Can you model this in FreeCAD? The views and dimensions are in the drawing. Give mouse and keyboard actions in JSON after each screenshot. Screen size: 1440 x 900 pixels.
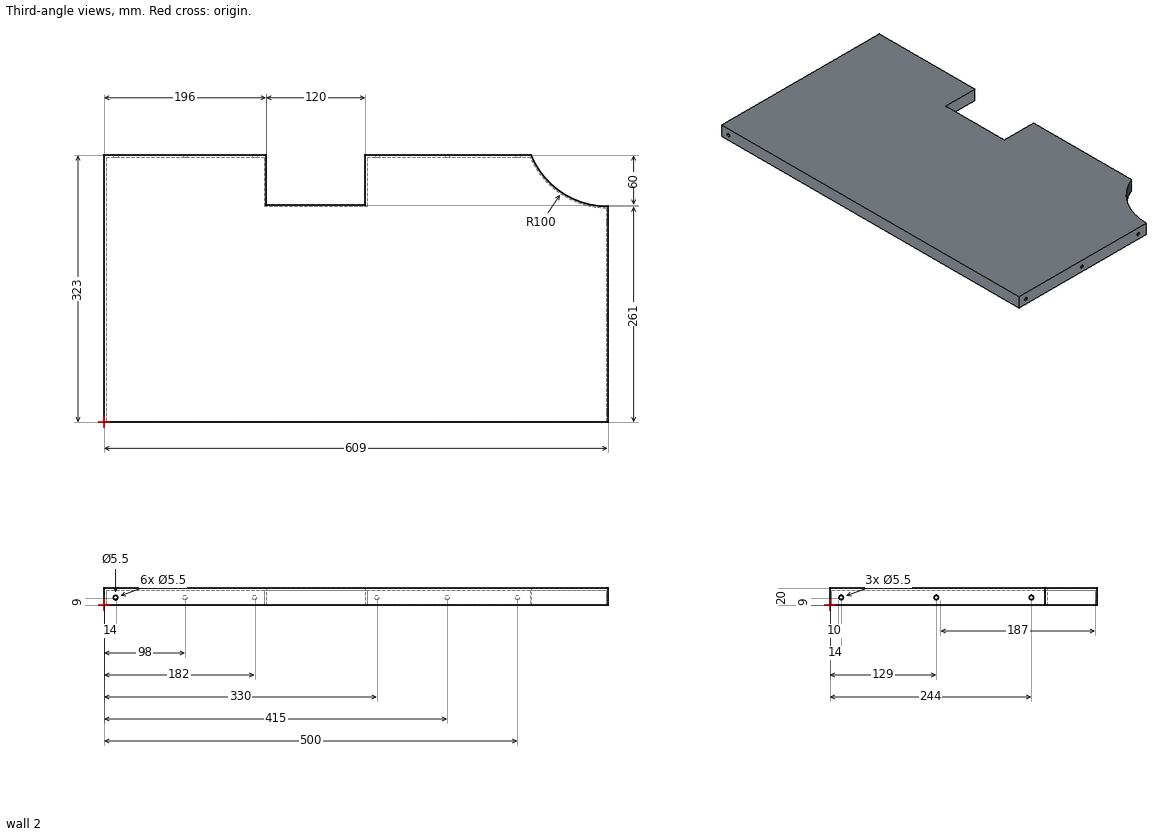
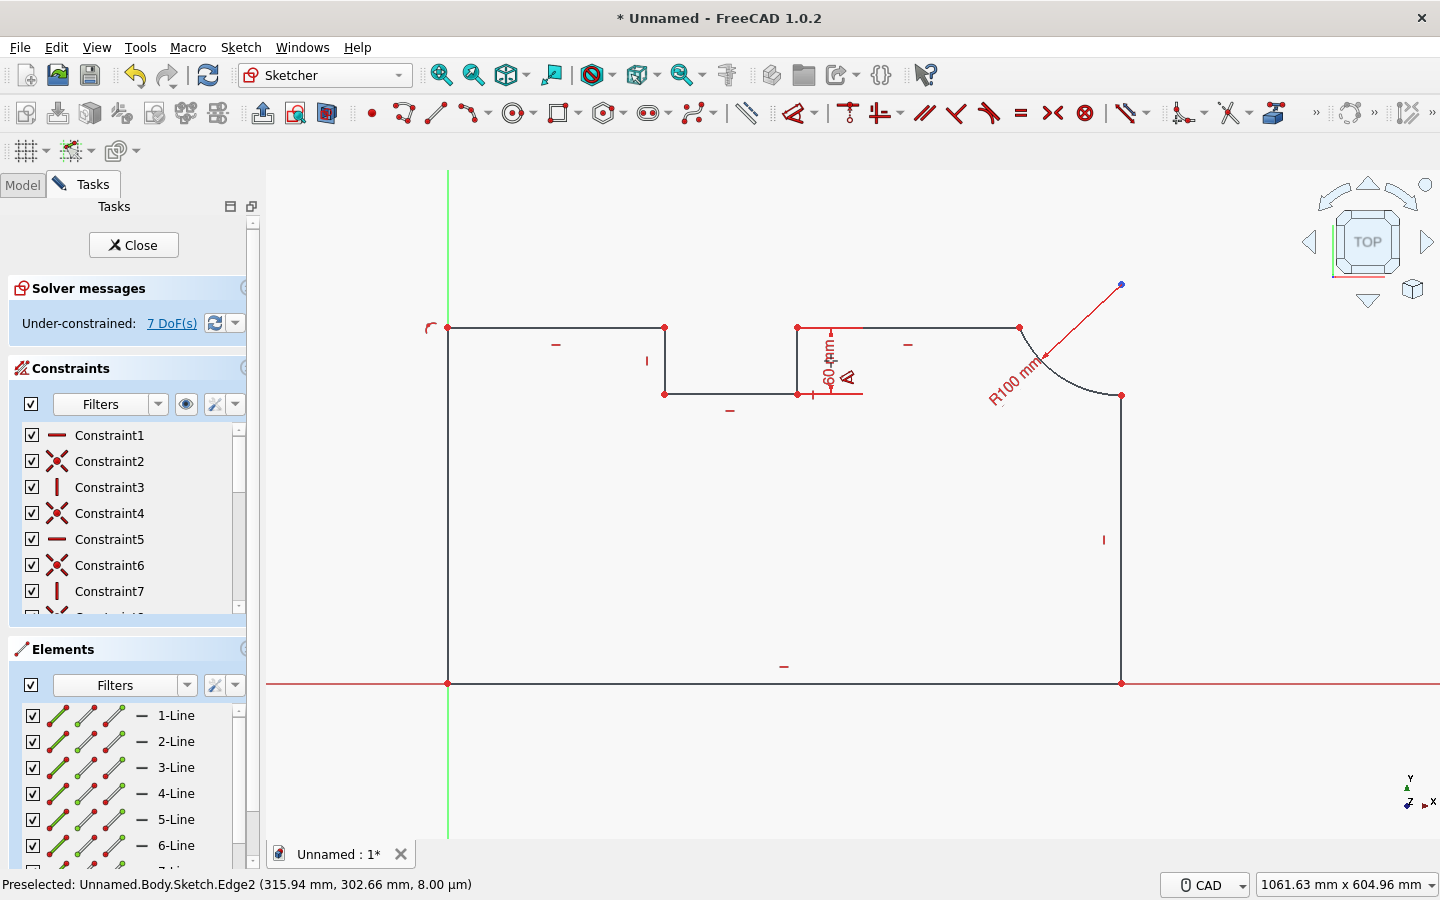
{"action": "left_click", "coordinate": [665, 374]}
{"action": "left_click", "coordinate": [631, 361]}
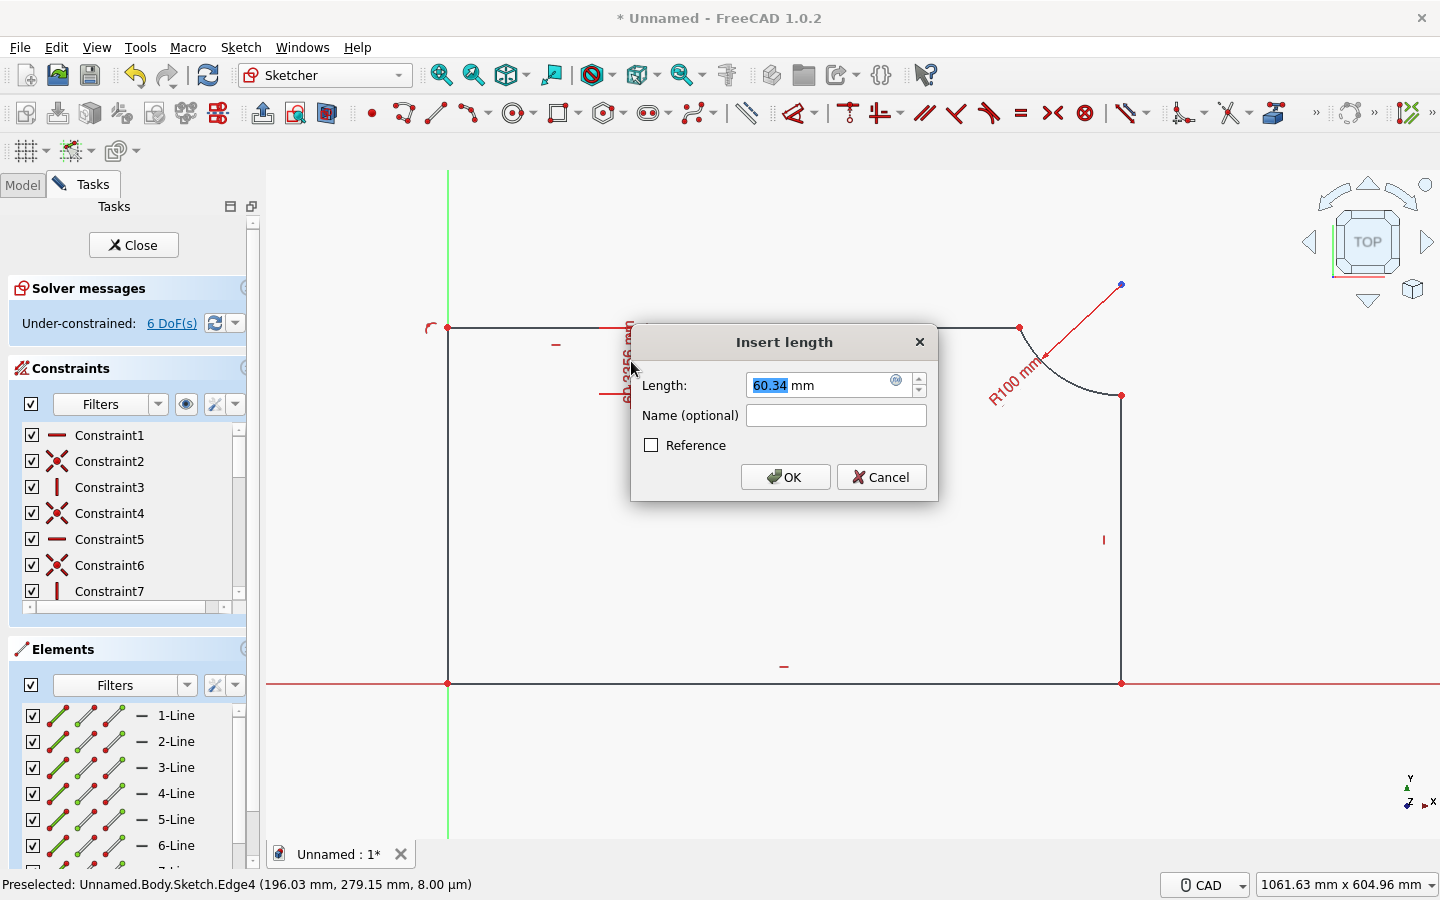
{"action": "type", "text": "60"}
{"action": "key", "text": "Return"}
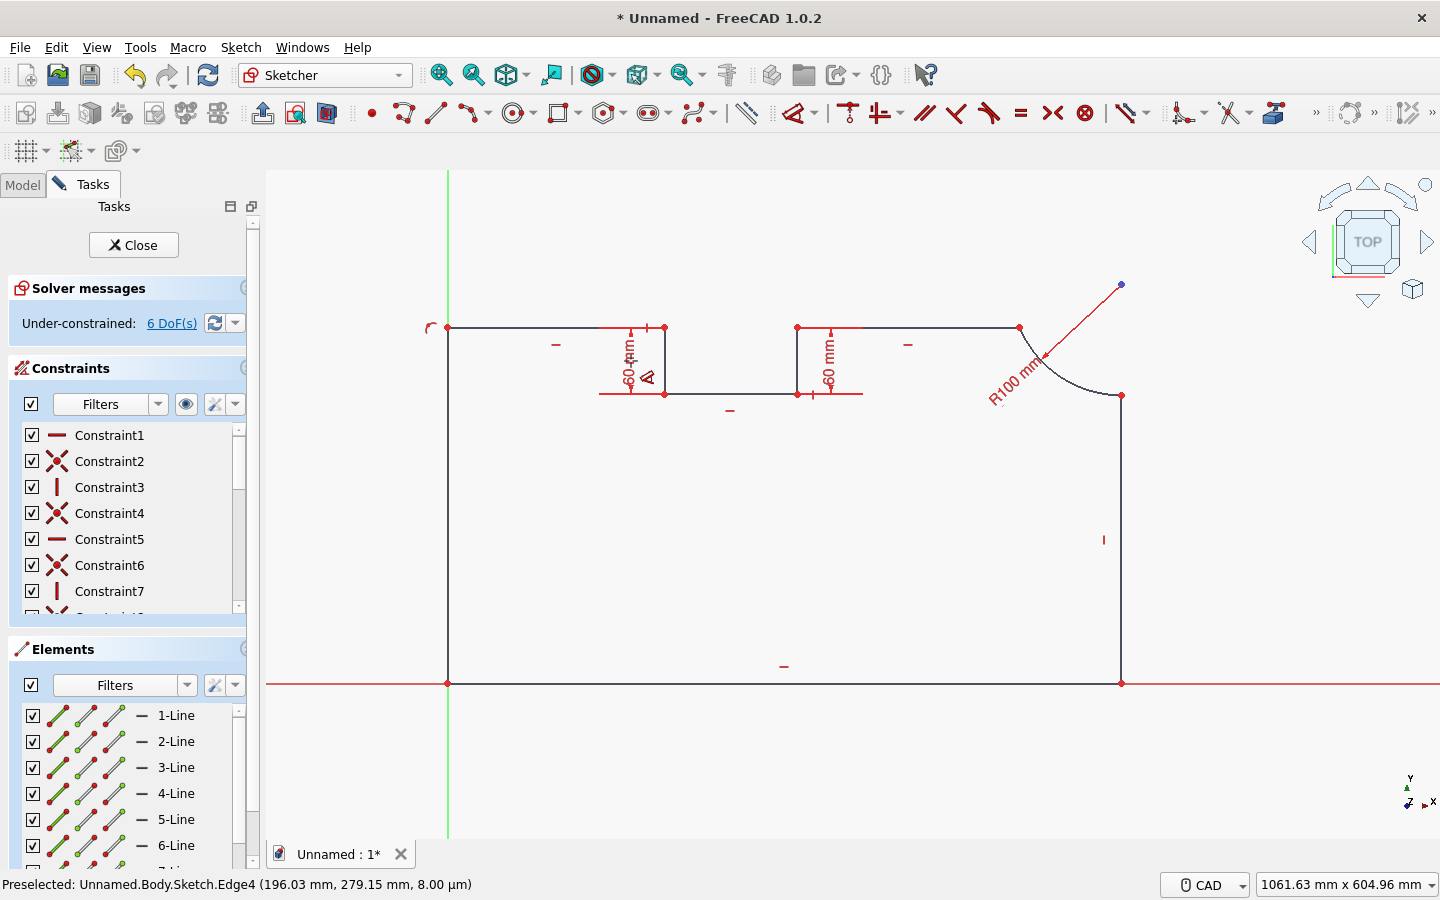
{"action": "left_click", "coordinate": [757, 394]}
{"action": "left_click", "coordinate": [731, 360]}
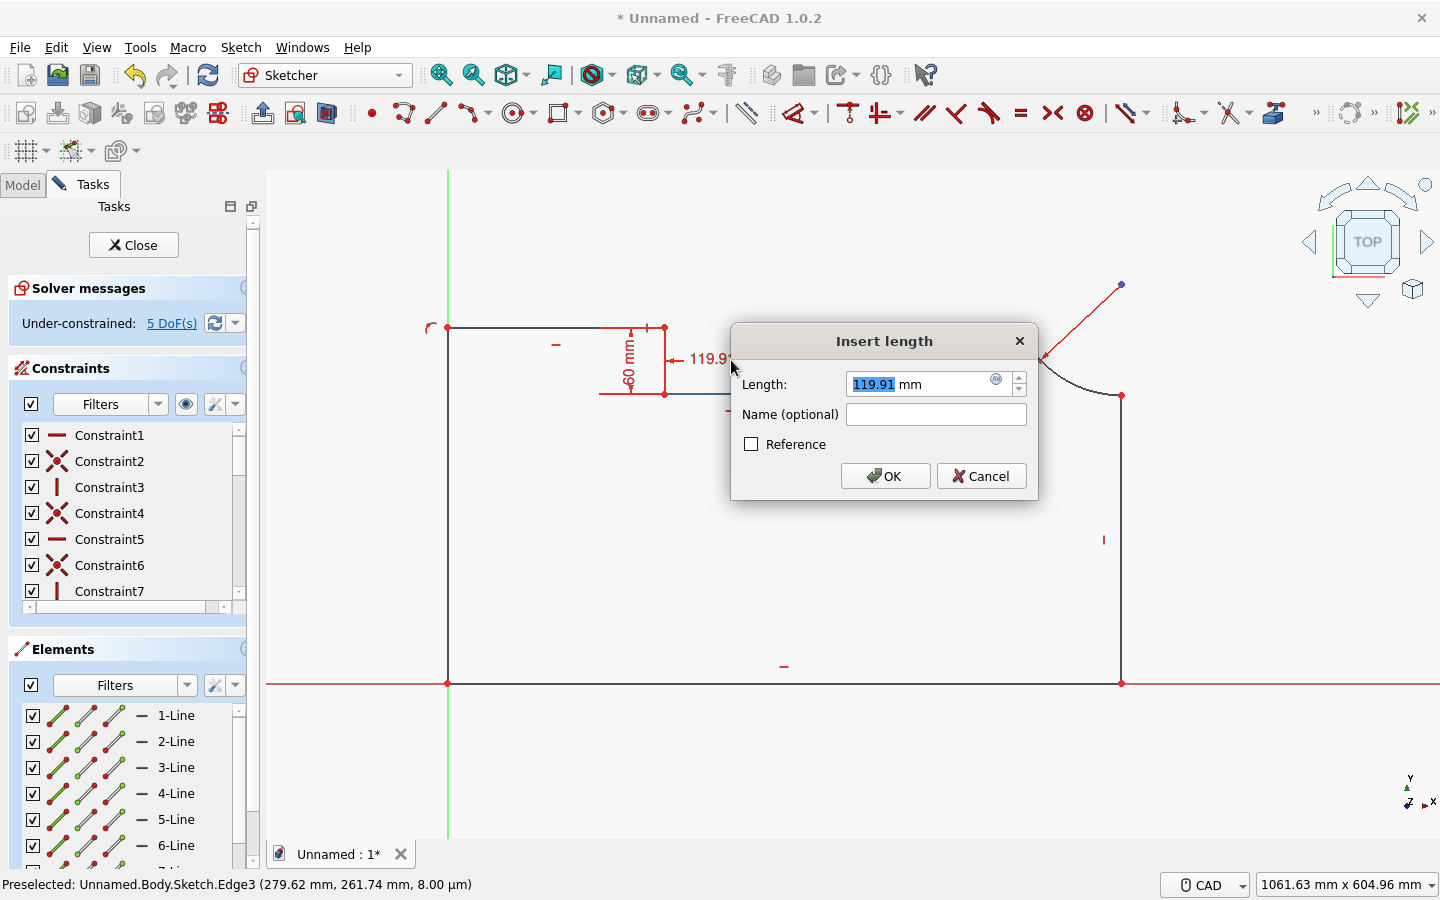
{"action": "type", "text": "120"}
{"action": "key", "text": "Return"}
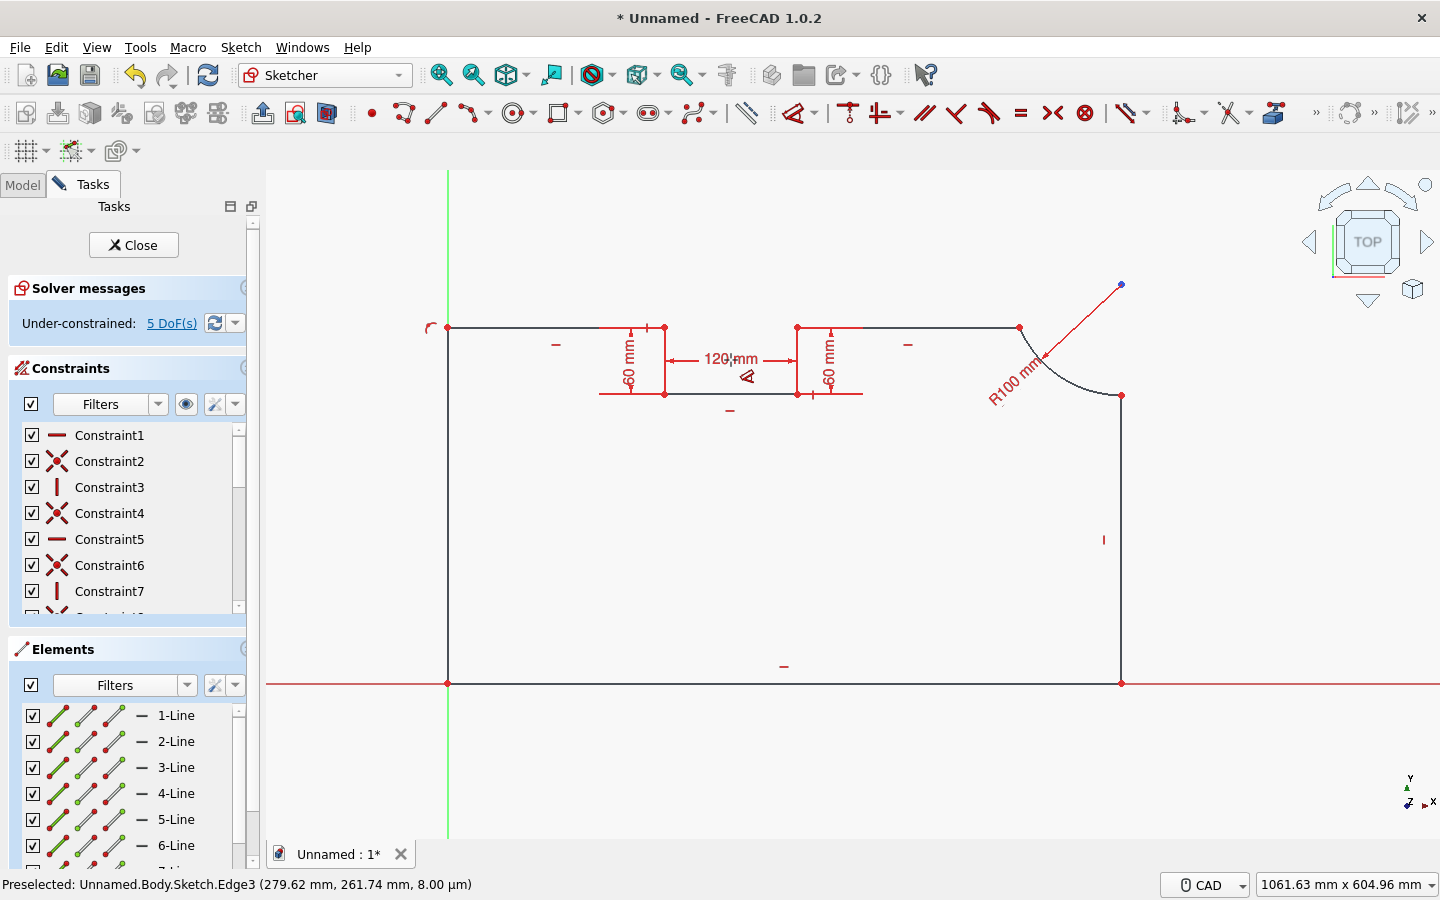
{"action": "left_click", "coordinate": [600, 328]}
{"action": "left_click", "coordinate": [556, 294]}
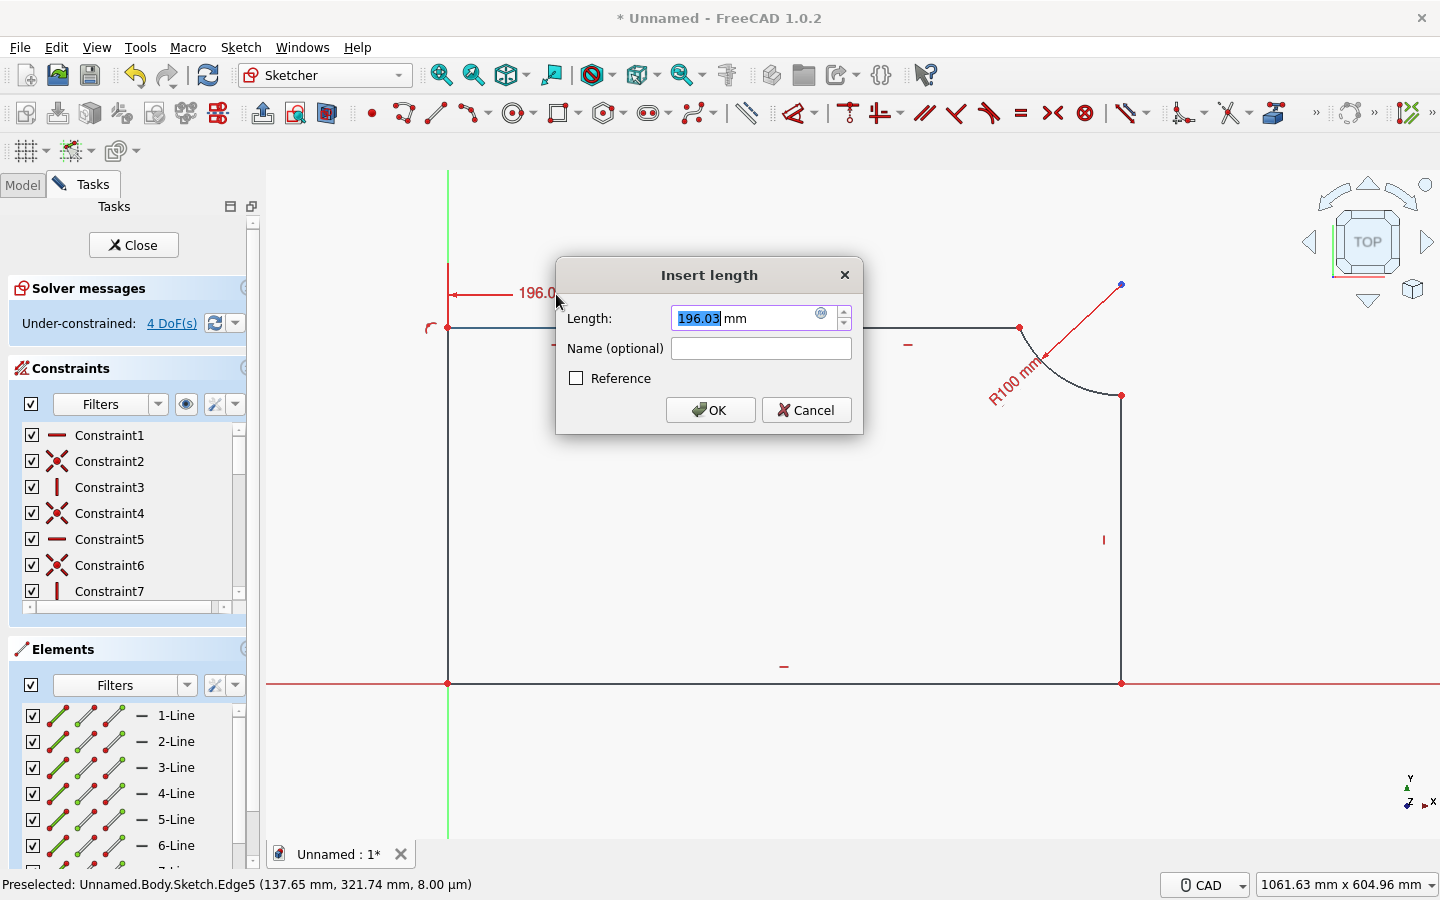
{"action": "type", "text": "196"}
{"action": "key", "text": "Return"}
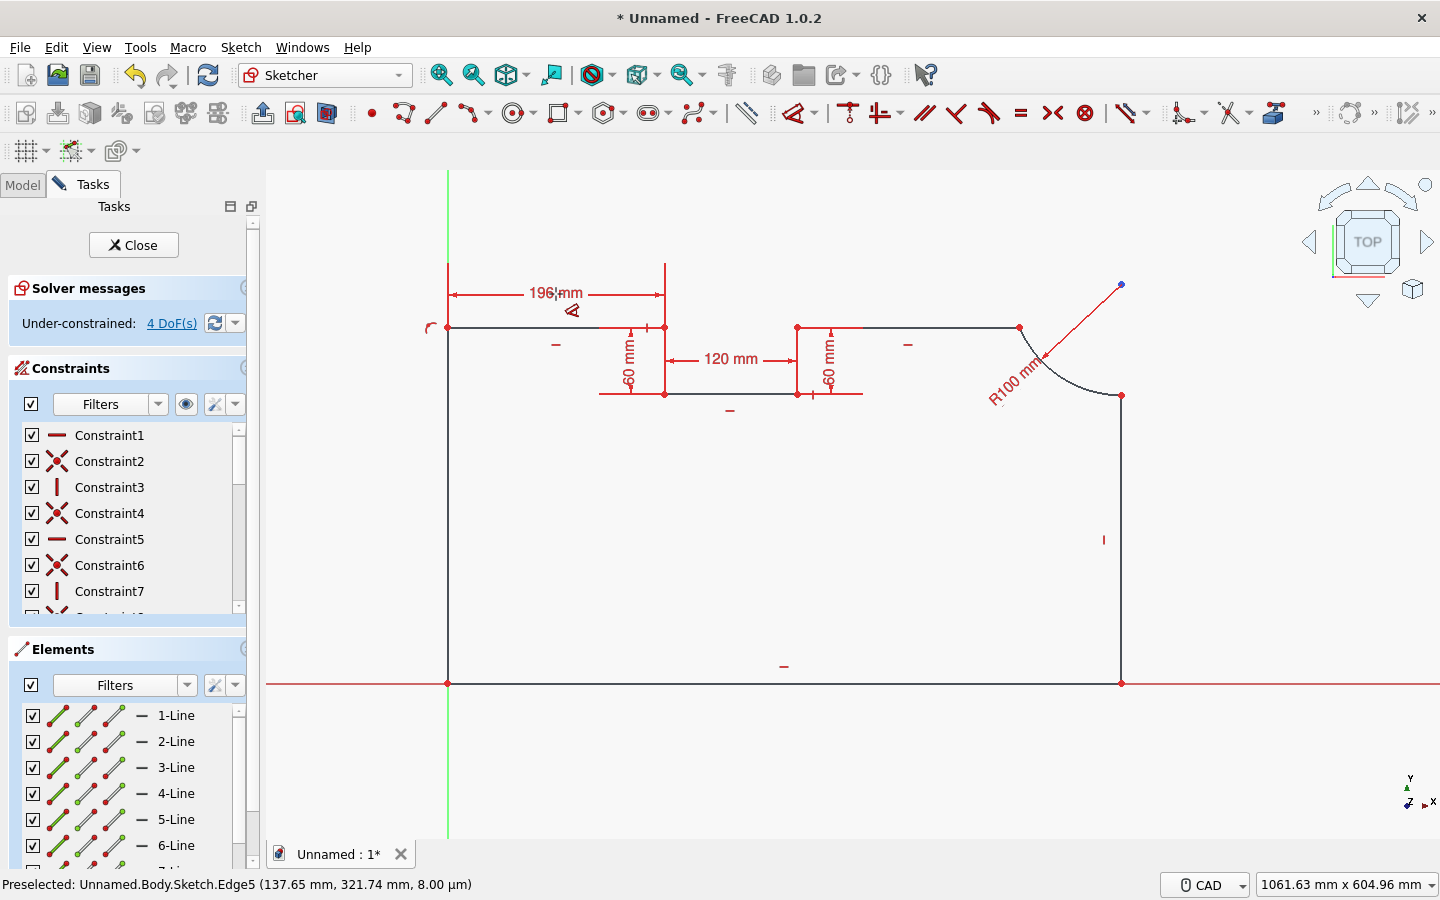
{"action": "left_click", "coordinate": [448, 435]}
{"action": "left_click", "coordinate": [414, 506]}